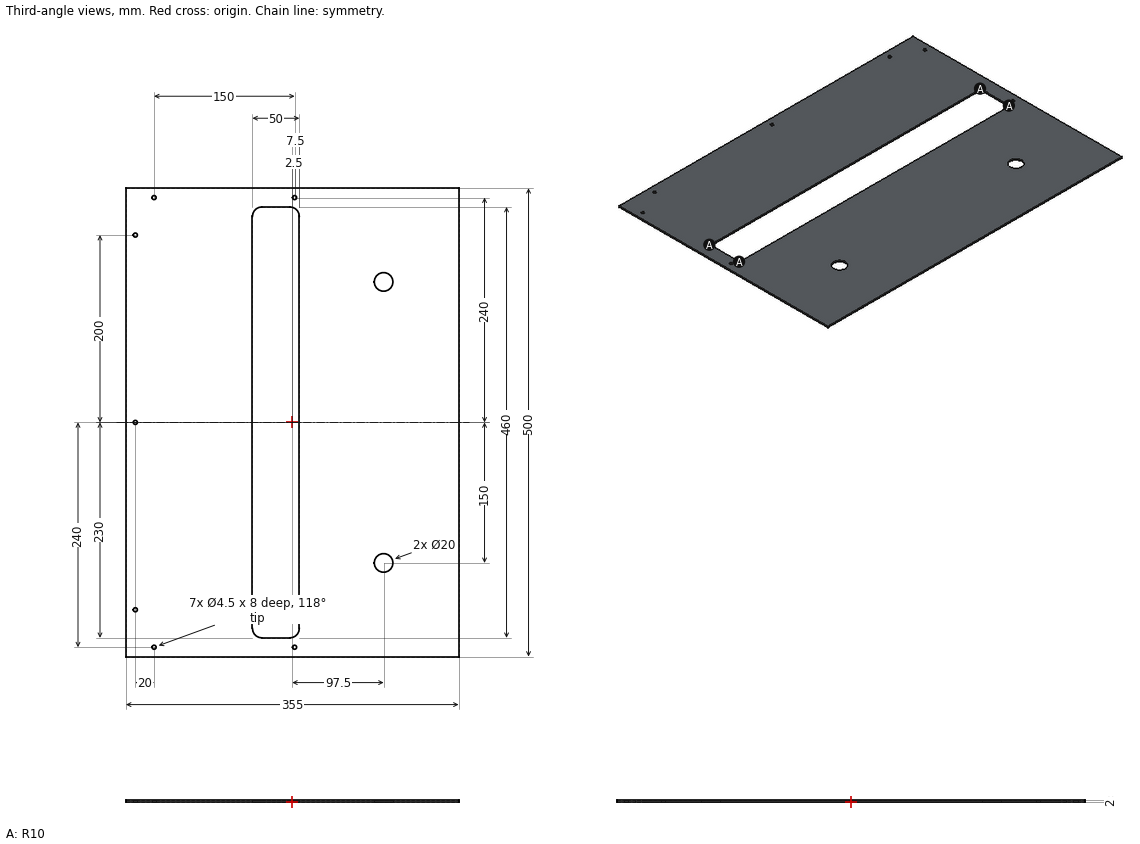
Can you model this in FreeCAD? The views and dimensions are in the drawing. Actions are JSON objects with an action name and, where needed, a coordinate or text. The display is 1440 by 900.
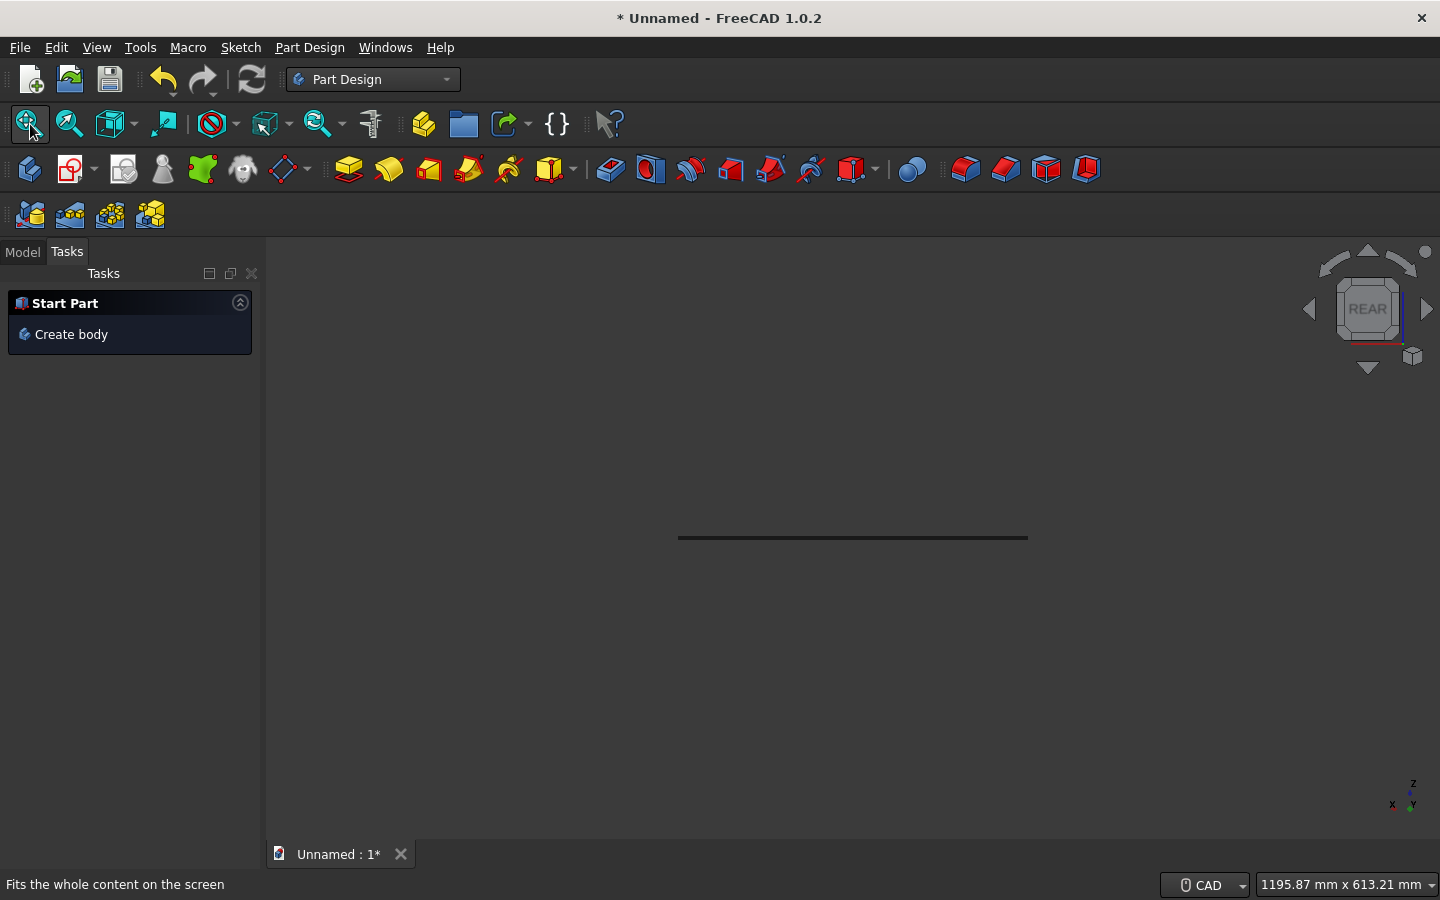
{"action": "key", "text": "6"}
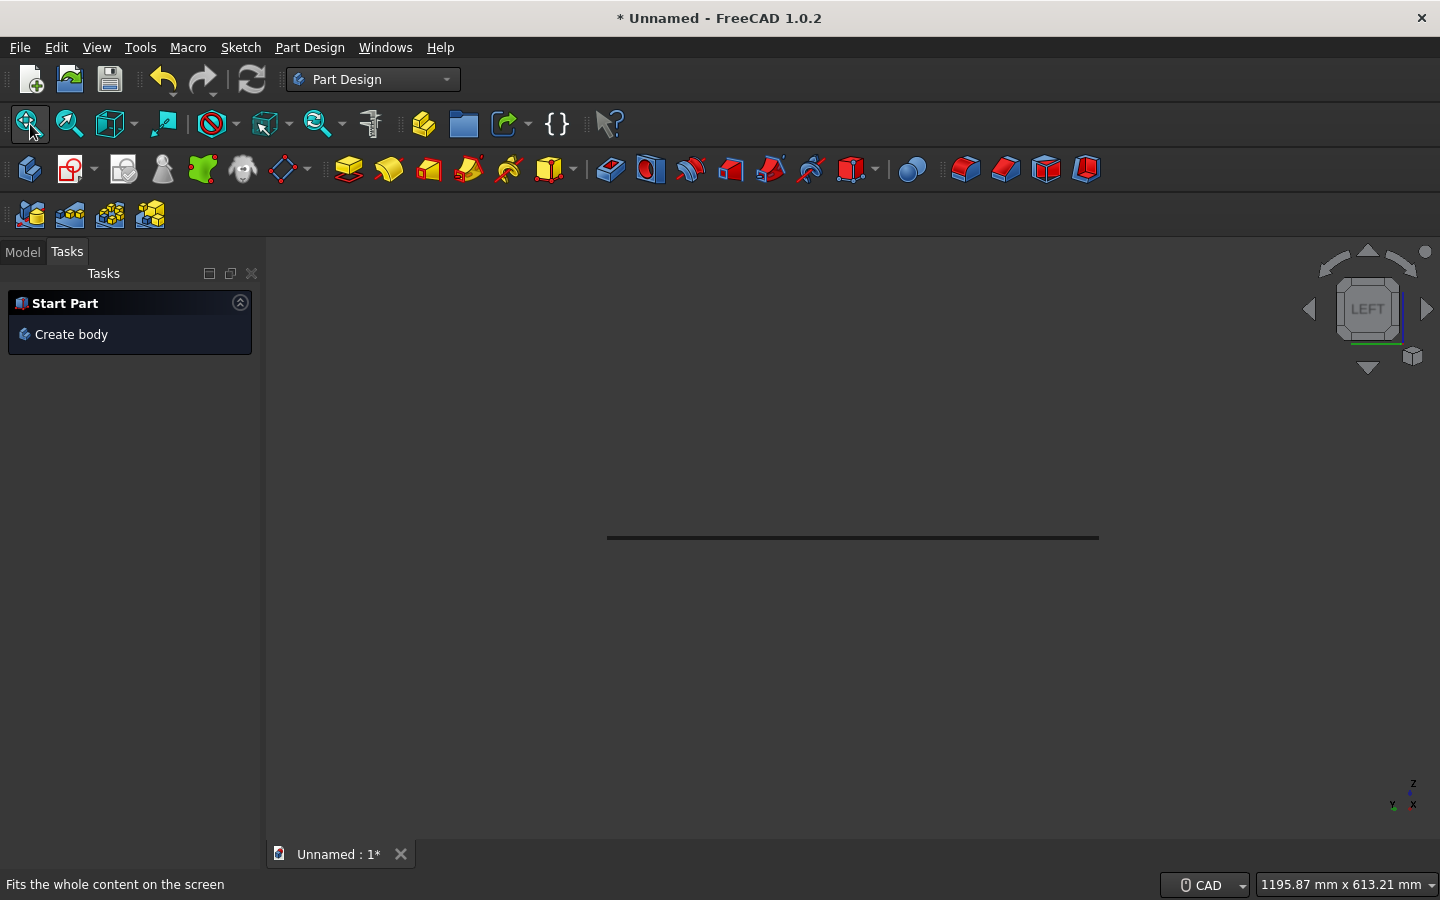
{"action": "left_click", "coordinate": [30, 124]}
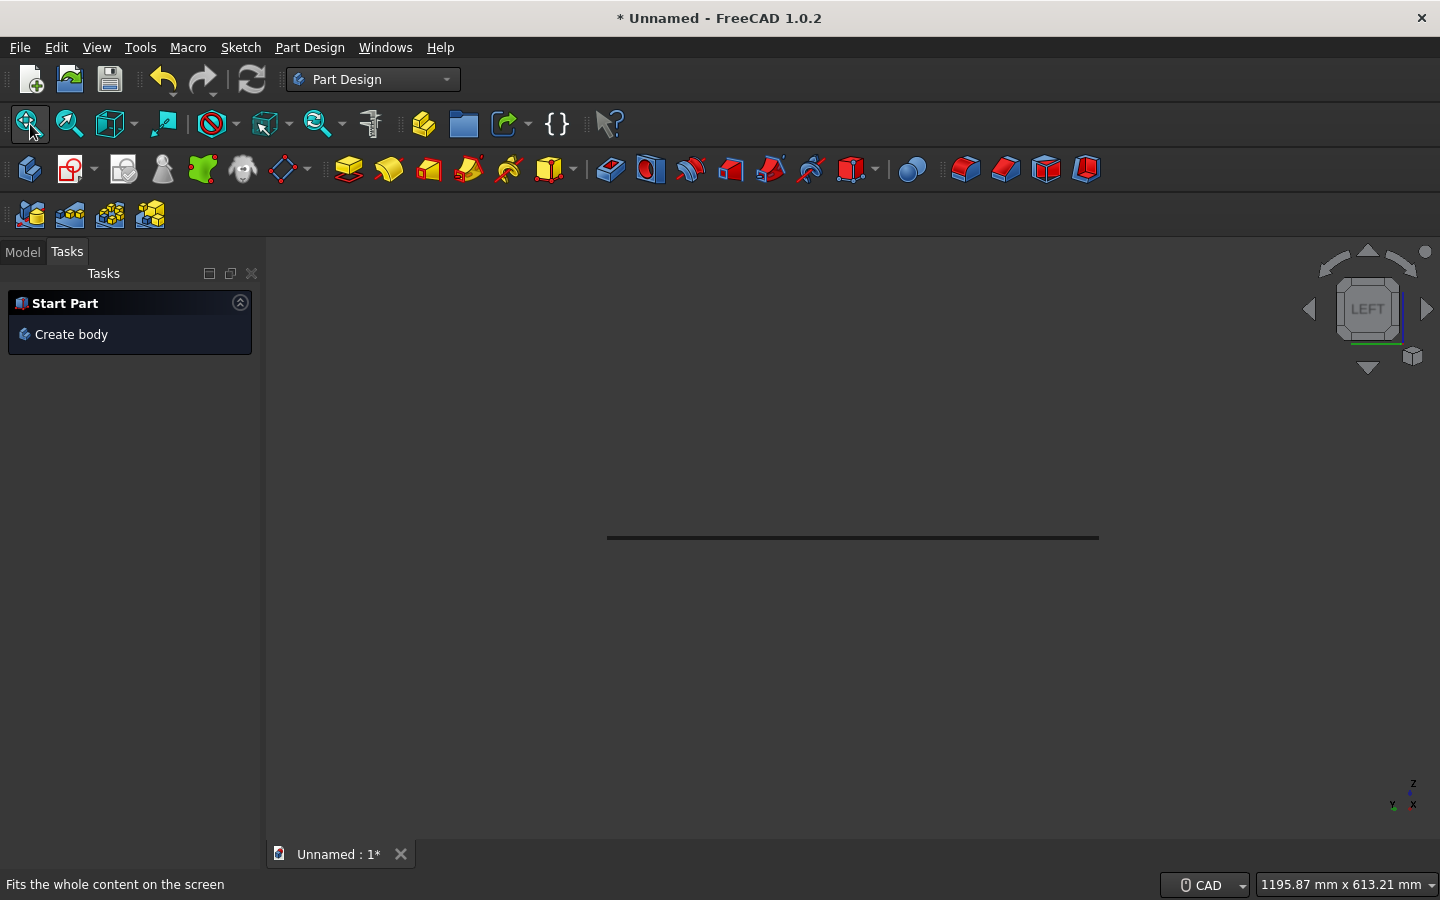
{"action": "scroll", "coordinate": [627, 537], "scroll_direction": "up", "scroll_amount": 15}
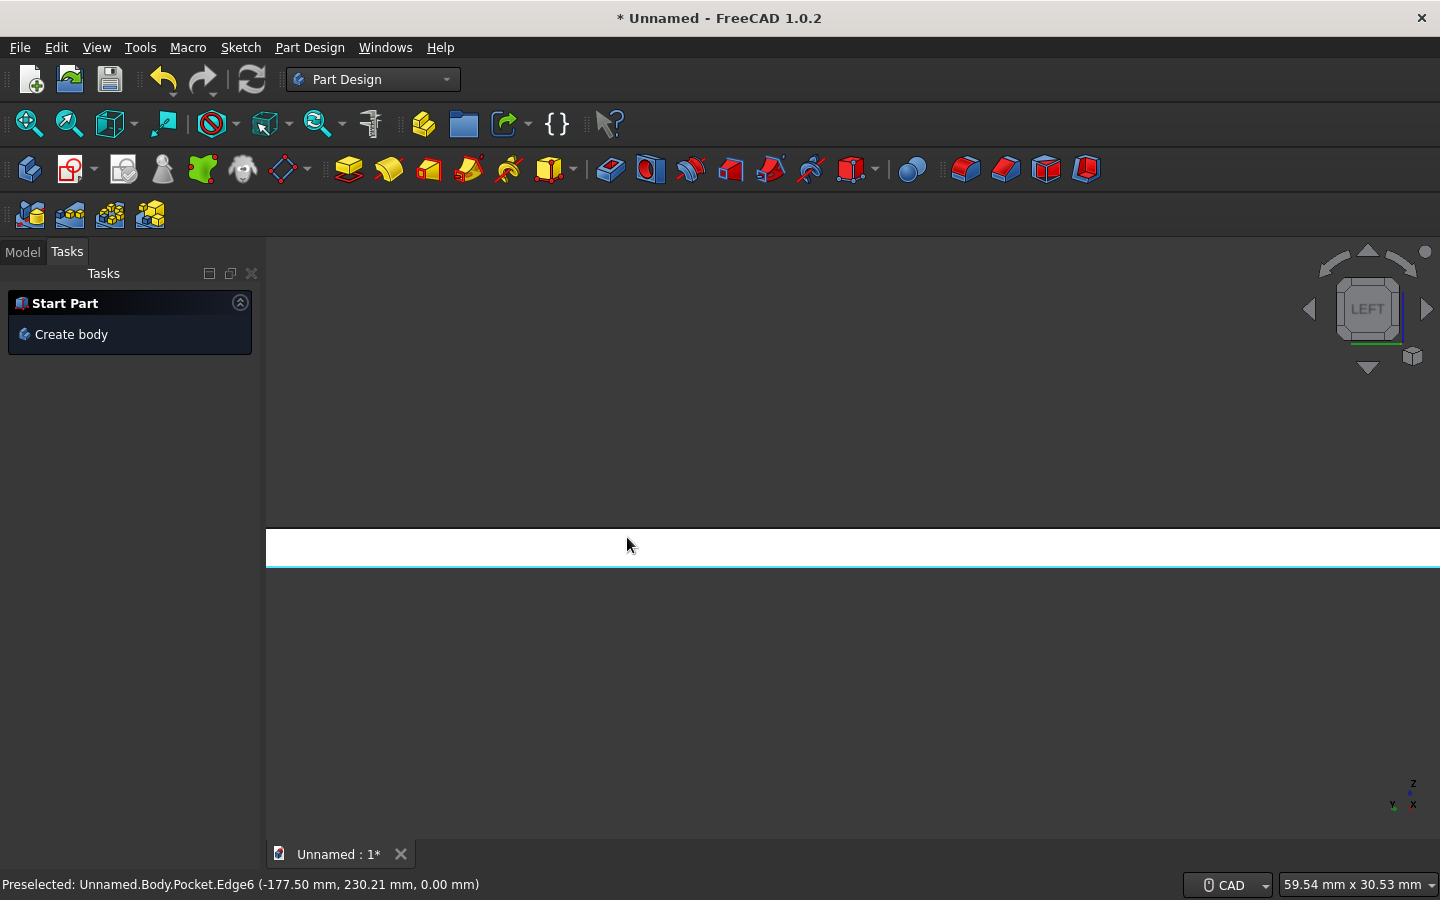
{"action": "left_click", "coordinate": [30, 124]}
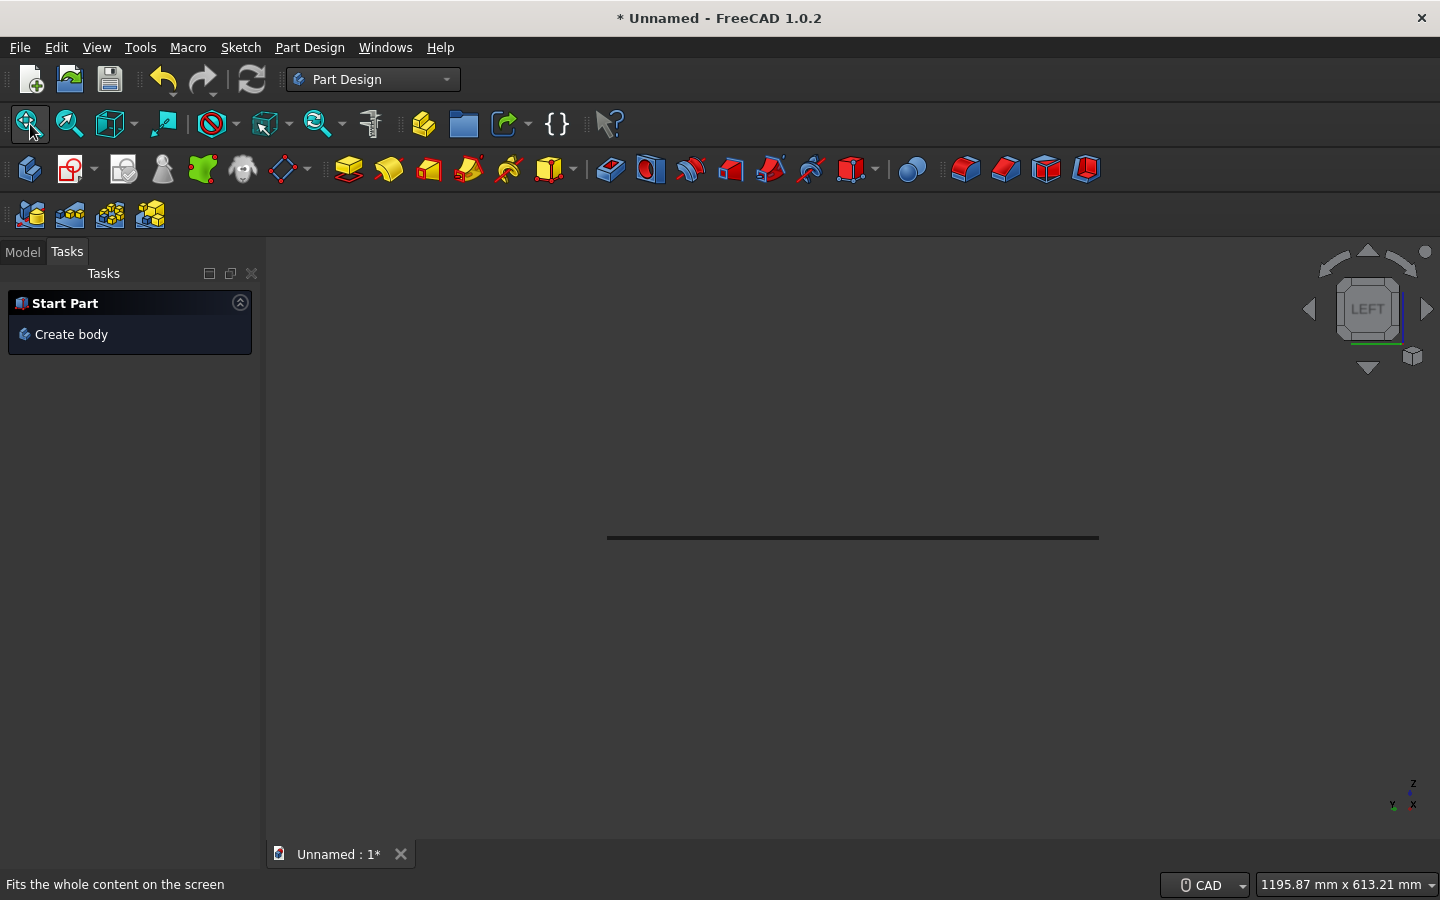
{"action": "key", "text": "v 3"}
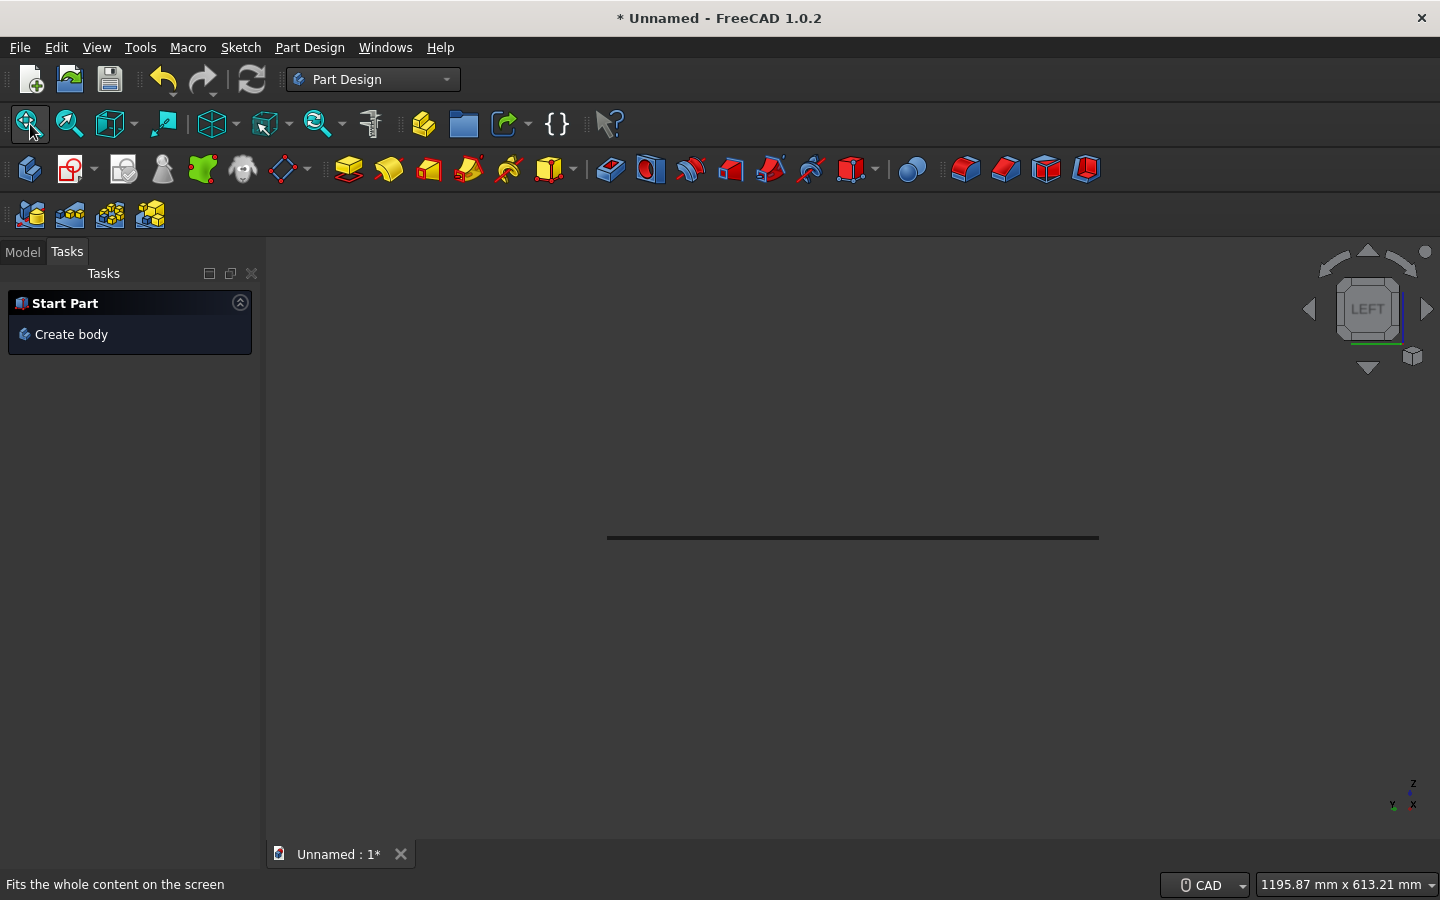
{"action": "key", "text": "0"}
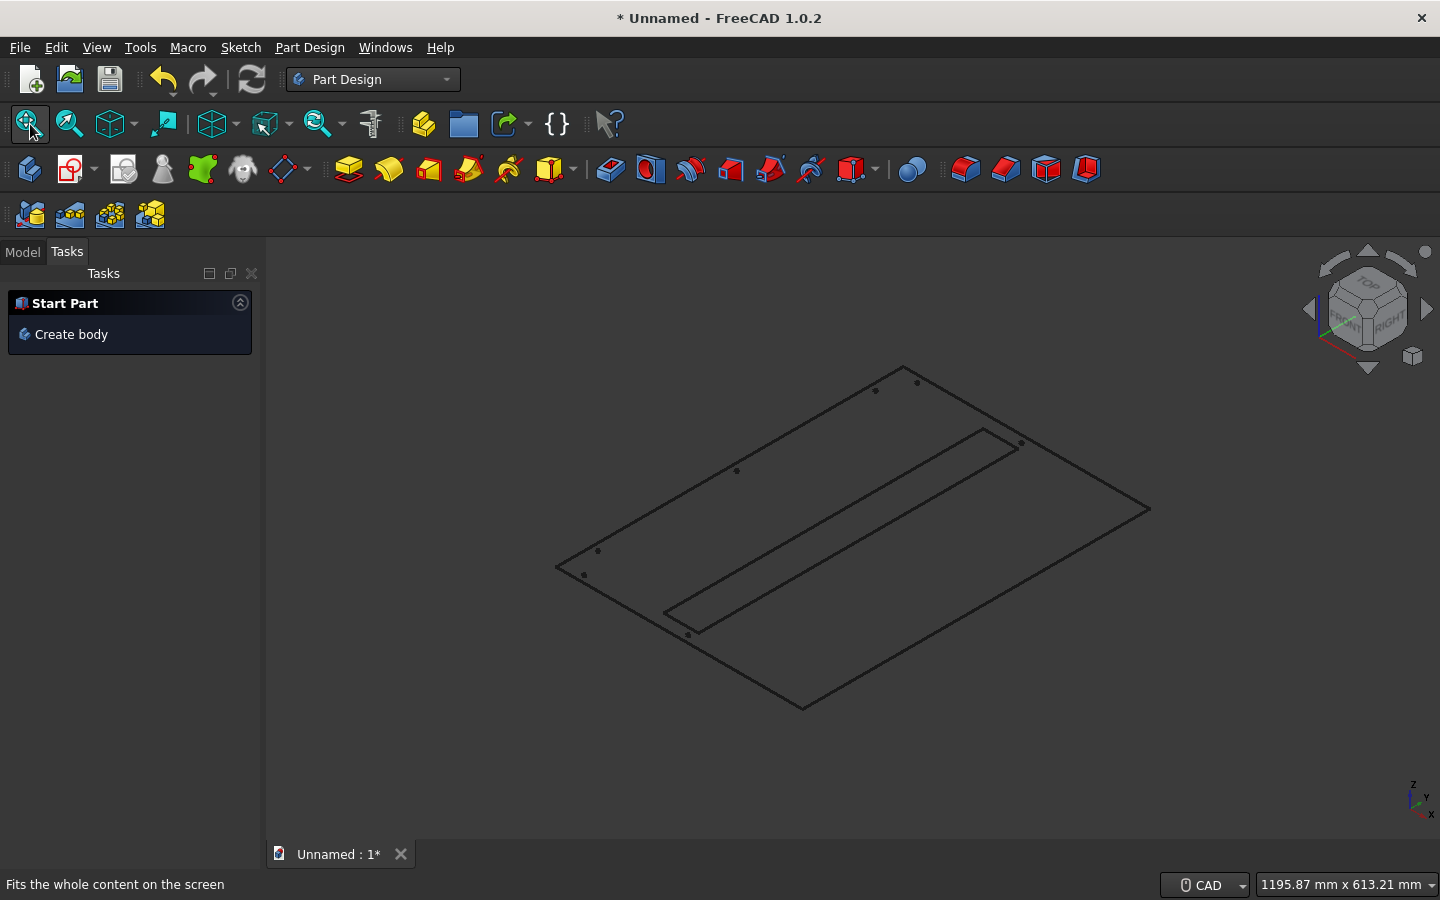
{"action": "scroll", "coordinate": [983, 428], "scroll_direction": "up", "scroll_amount": 15}